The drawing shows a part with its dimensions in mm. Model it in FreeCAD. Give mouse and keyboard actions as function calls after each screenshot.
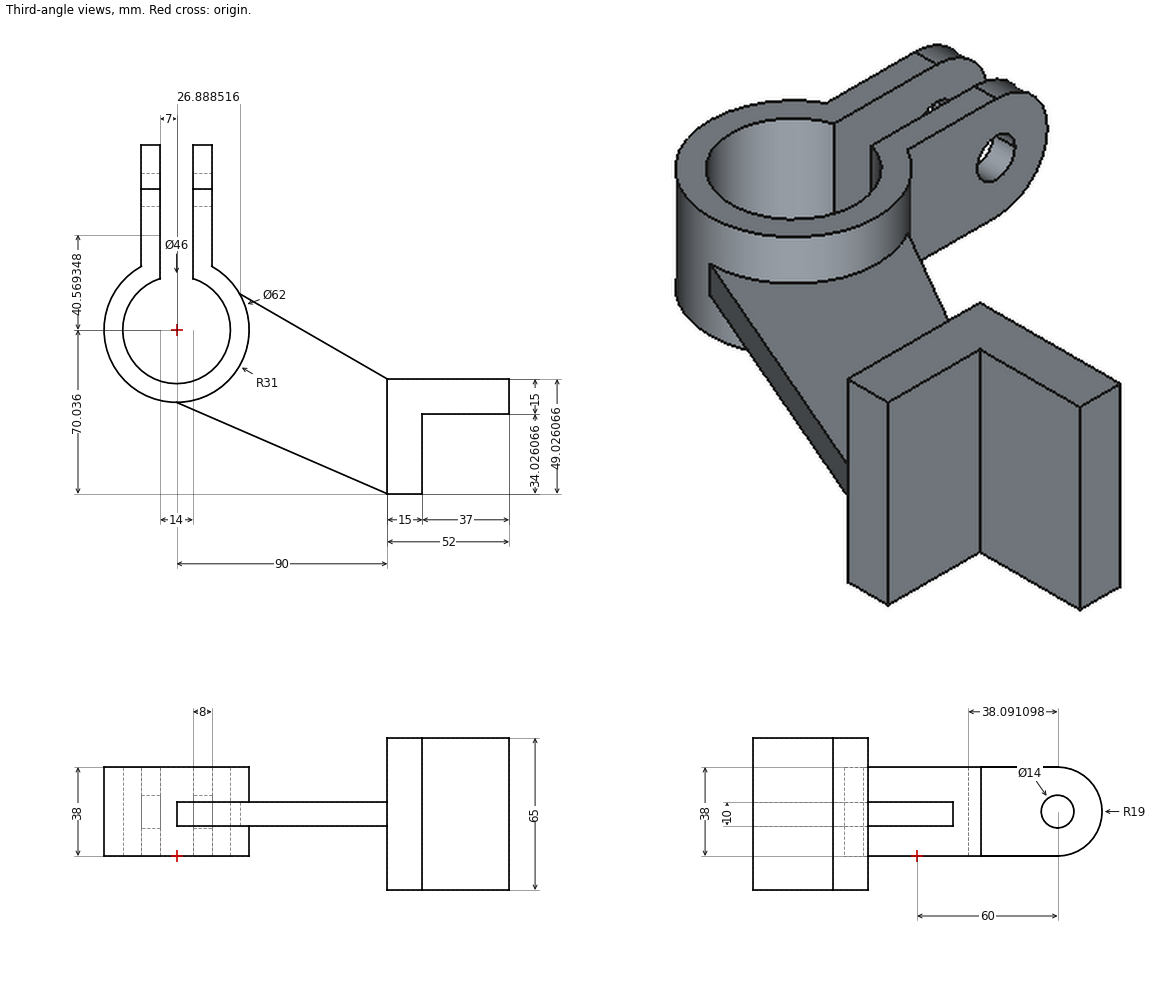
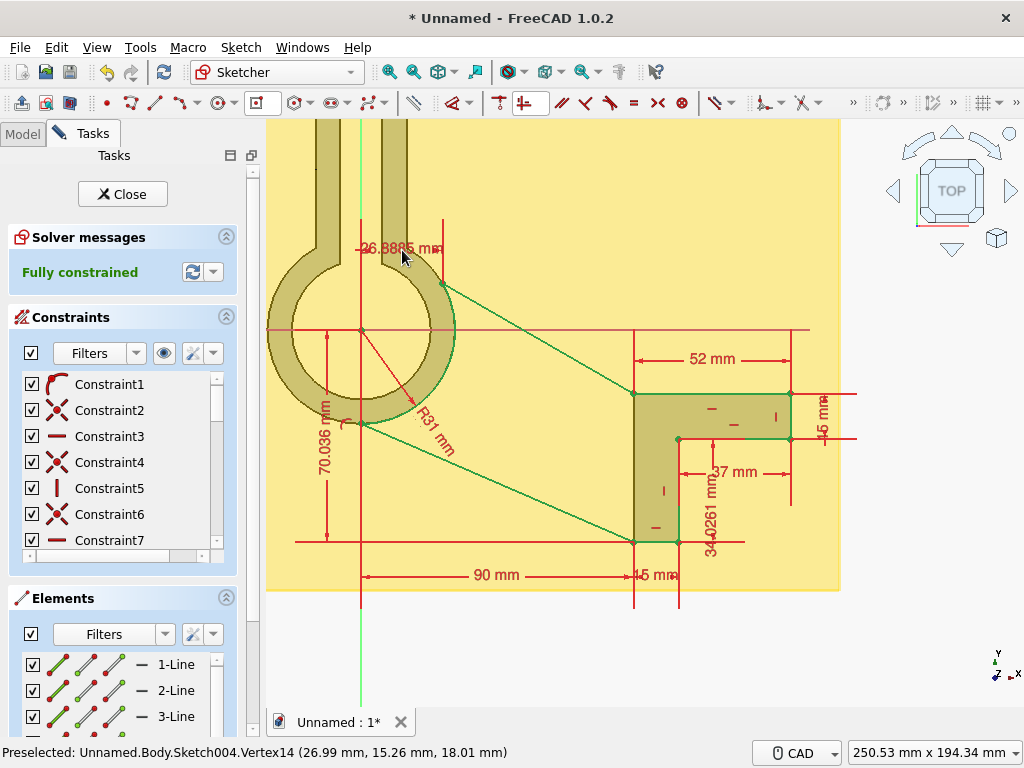
click(123, 194)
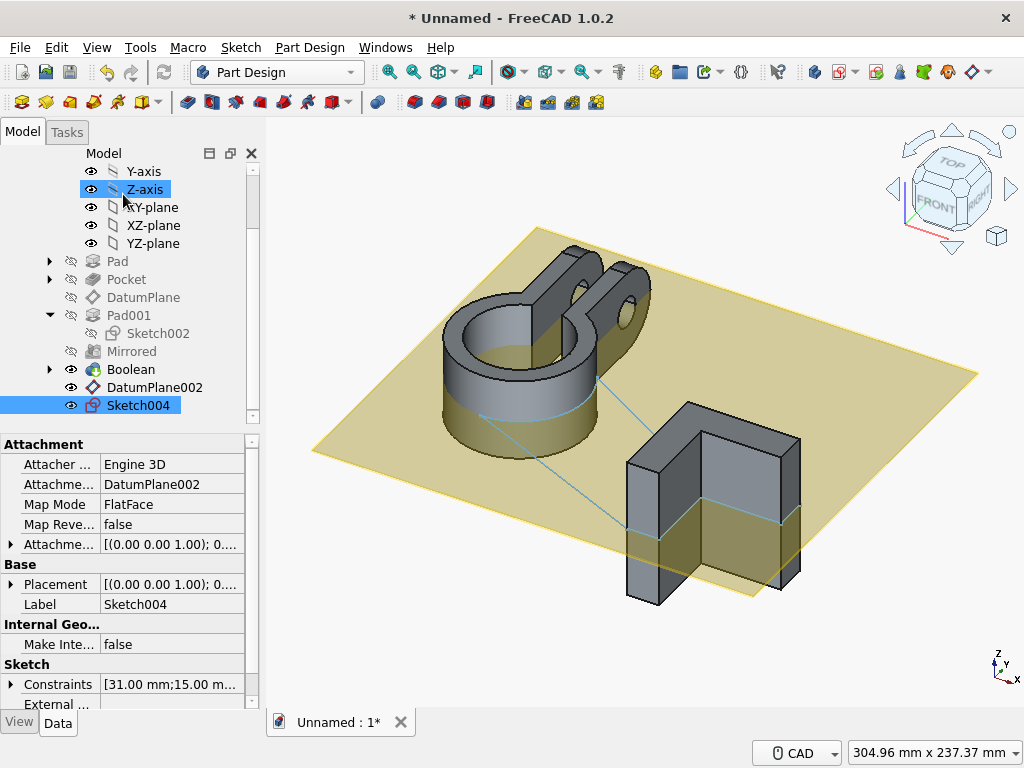
click(22, 102)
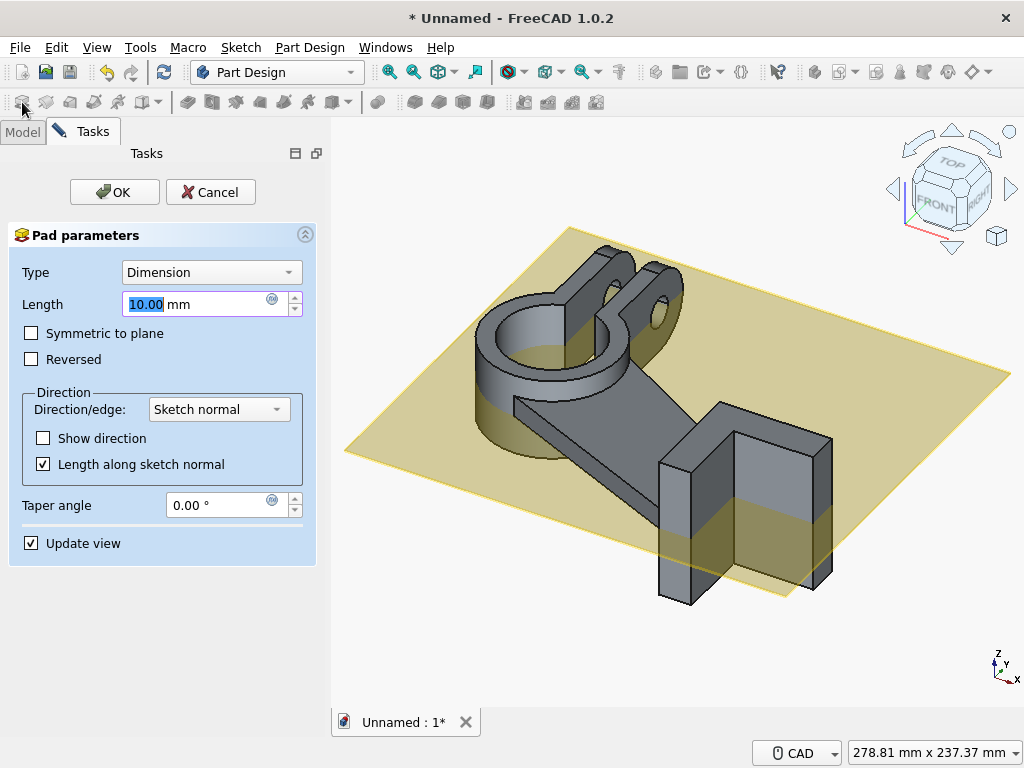
text(10)
key(Tab)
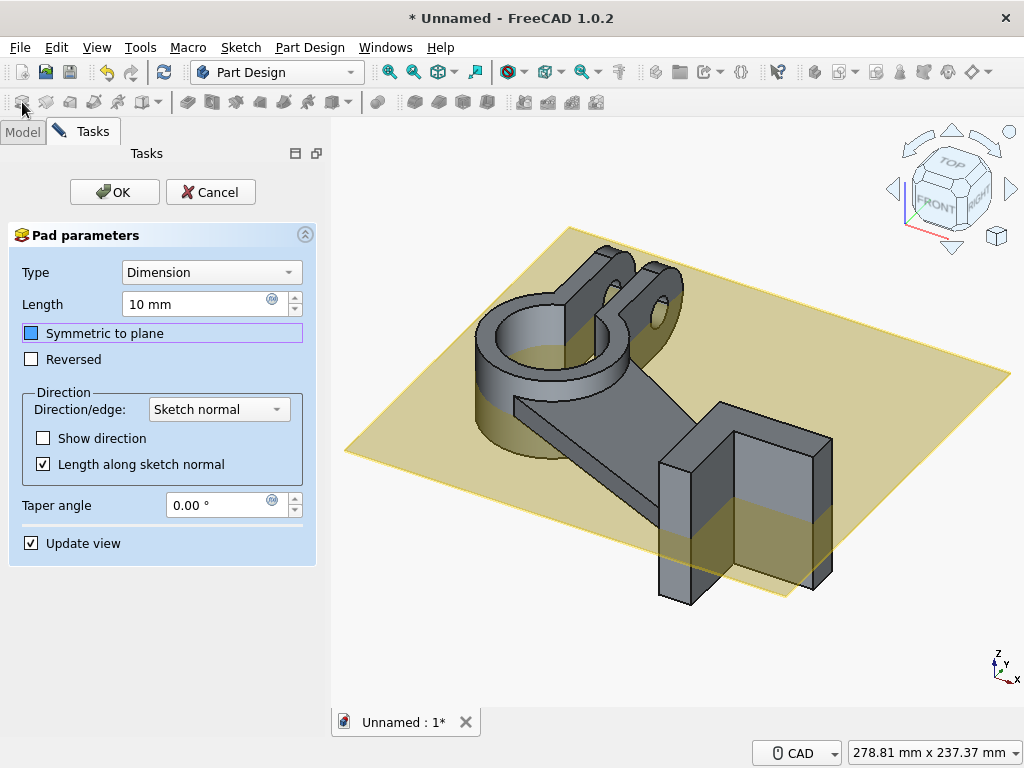
click(30, 333)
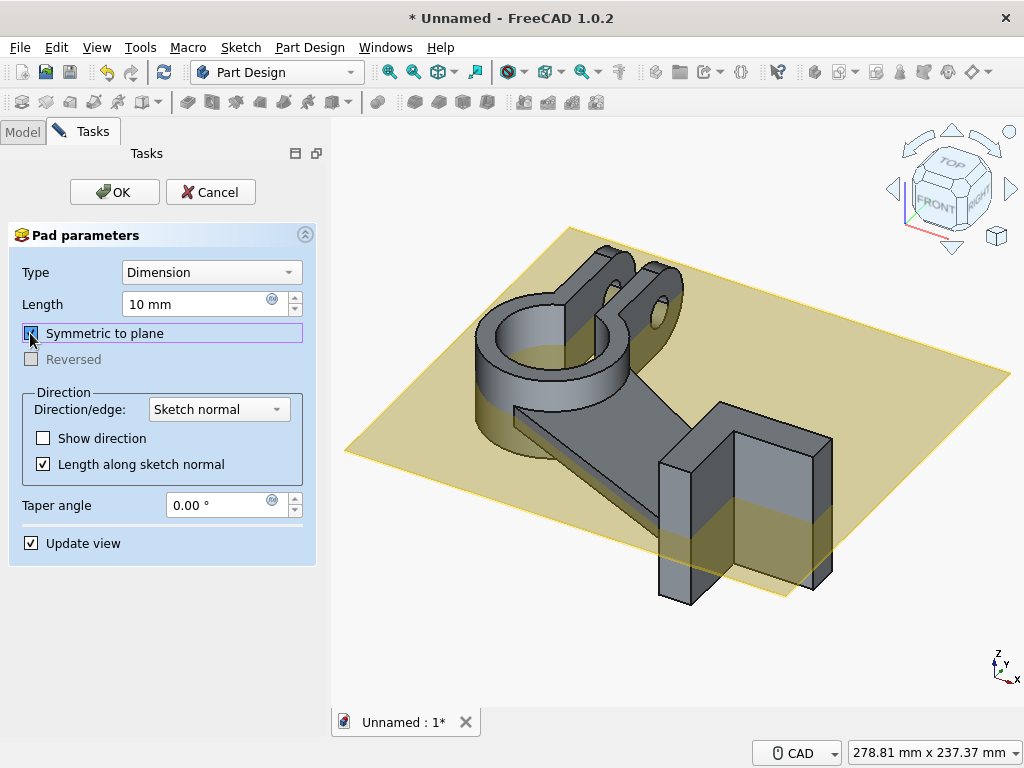
click(115, 192)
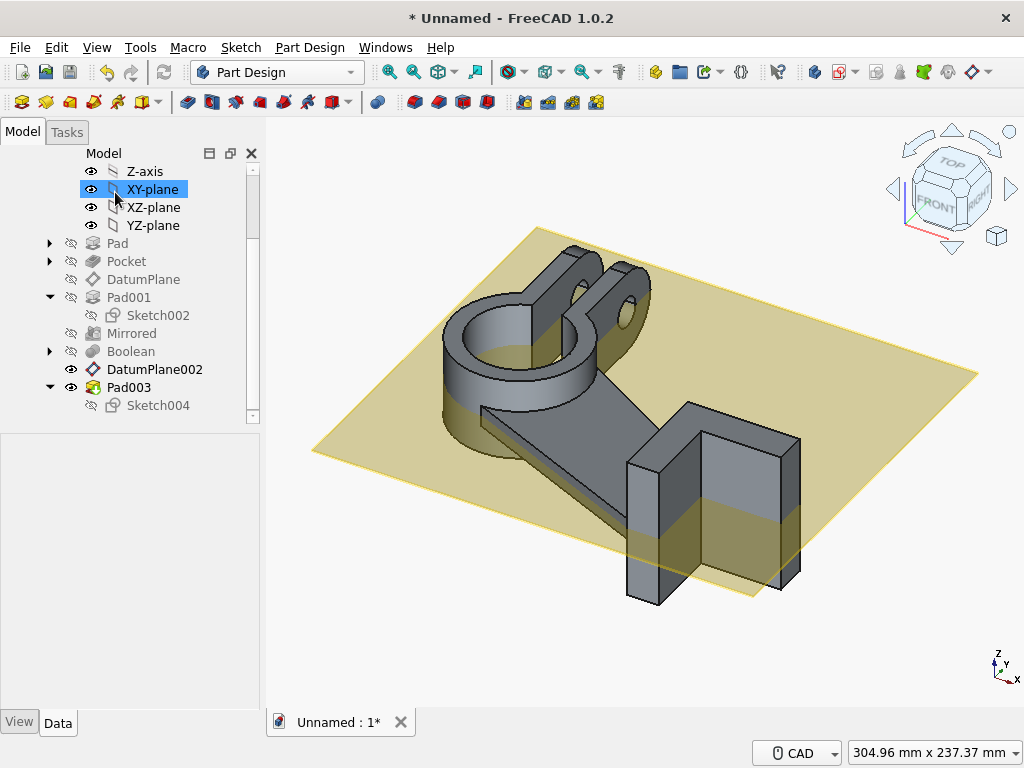
click(116, 369)
key(space)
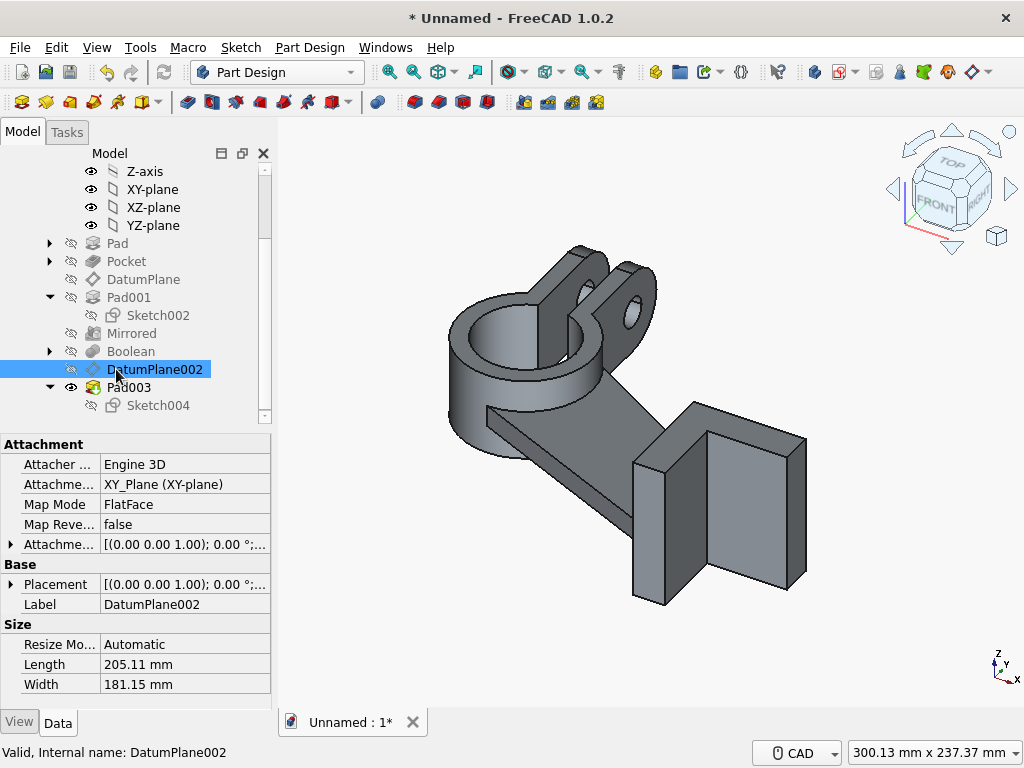
key(0)